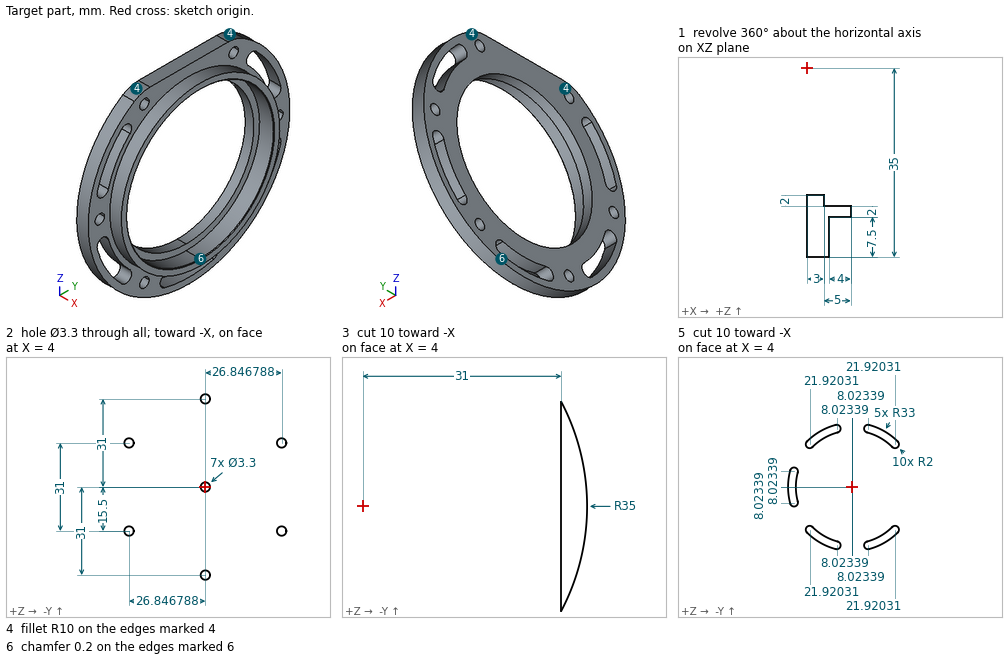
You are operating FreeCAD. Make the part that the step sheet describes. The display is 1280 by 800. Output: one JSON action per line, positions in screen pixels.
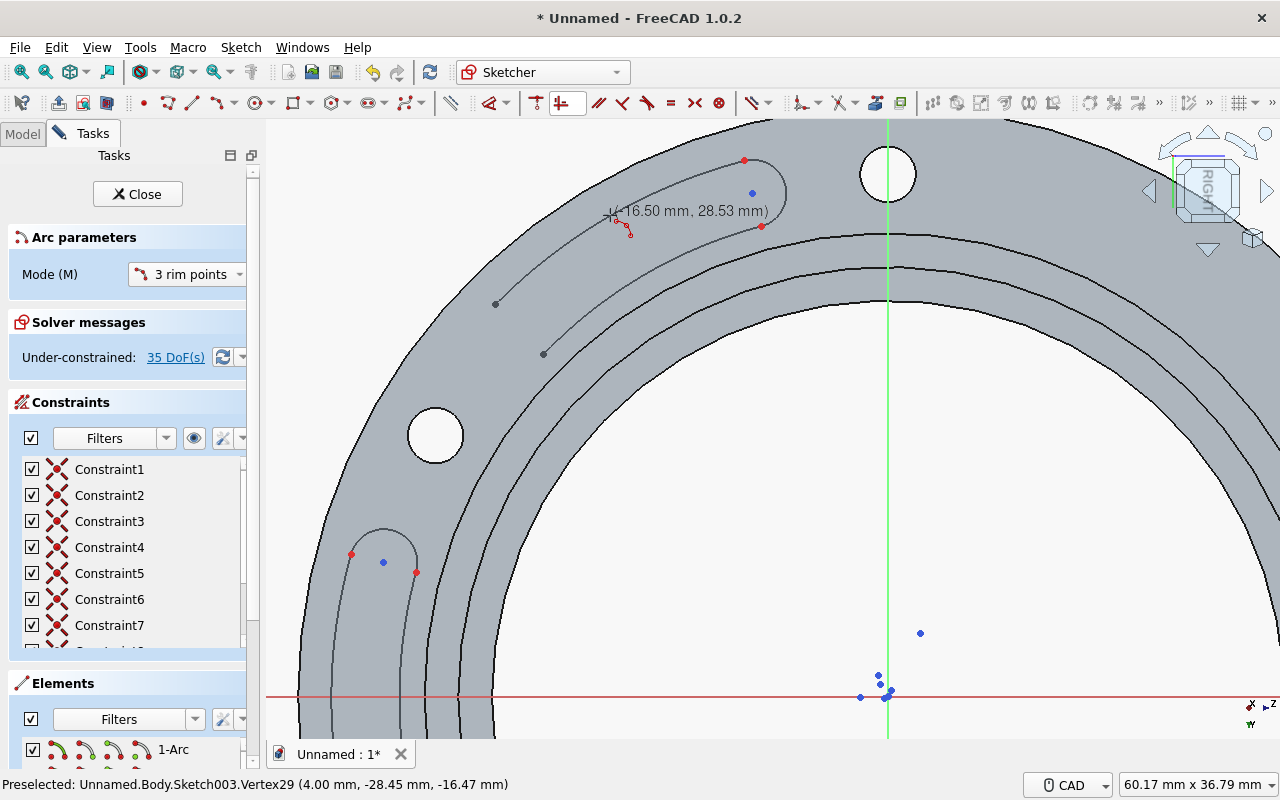
{"action": "left_click", "coordinate": [495, 305]}
{"action": "left_click", "coordinate": [544, 354]}
{"action": "left_click", "coordinate": [495, 351]}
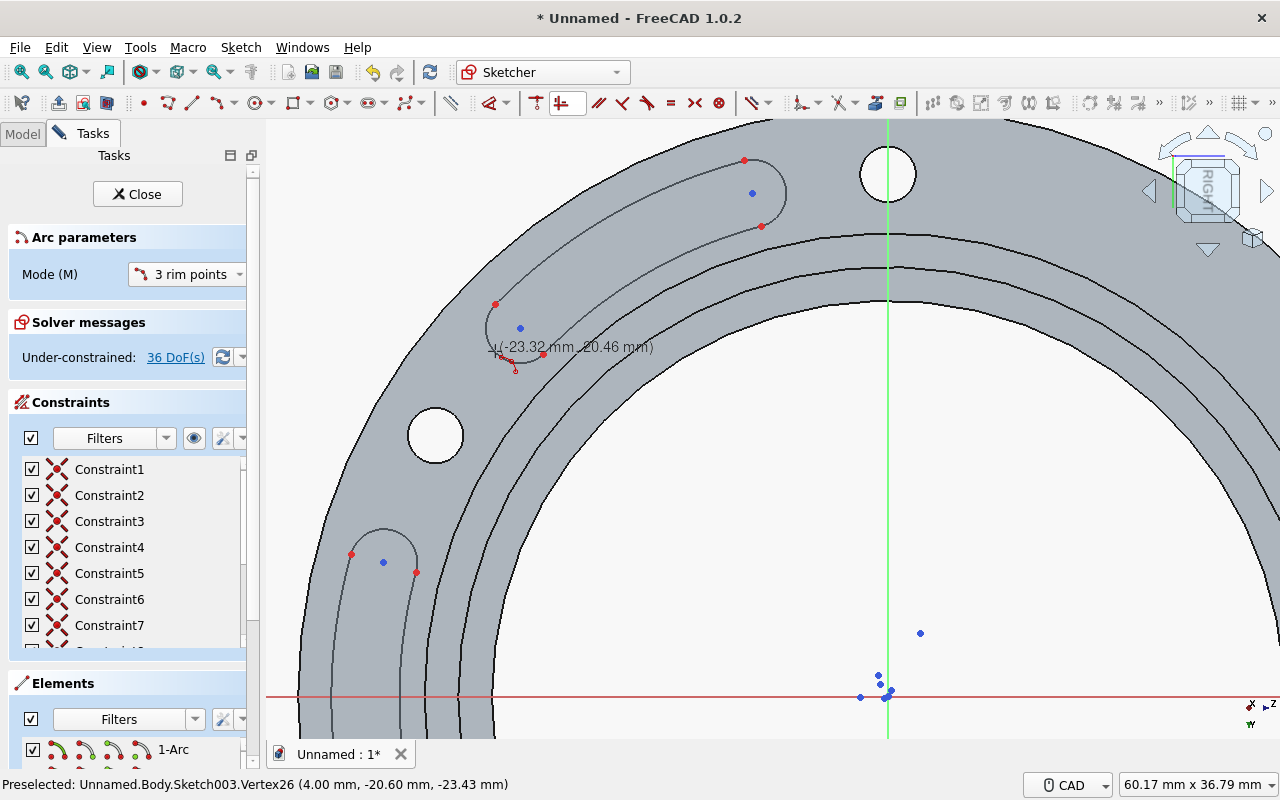
{"action": "scroll", "coordinate": [645, 273], "scroll_direction": "down", "scroll_amount": 5}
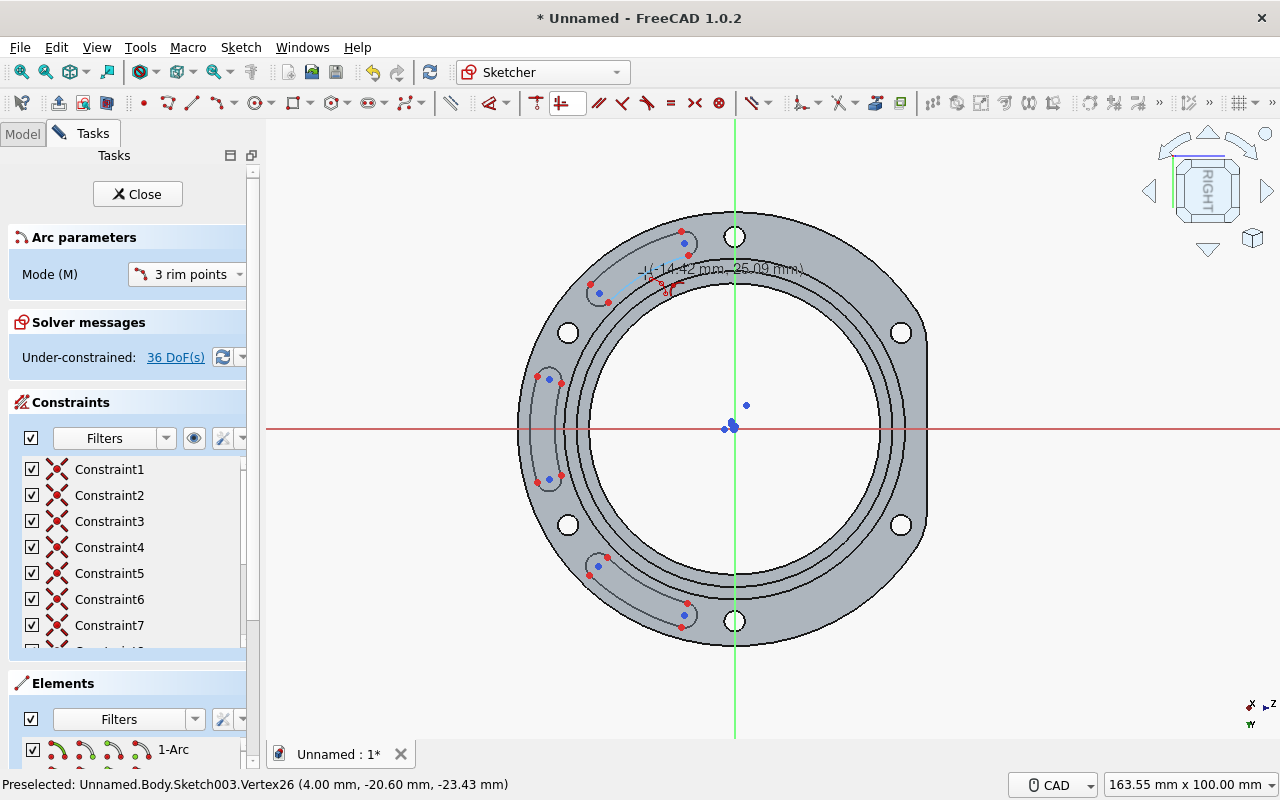
{"action": "left_click", "coordinate": [862, 302]}
{"action": "left_click", "coordinate": [879, 284]}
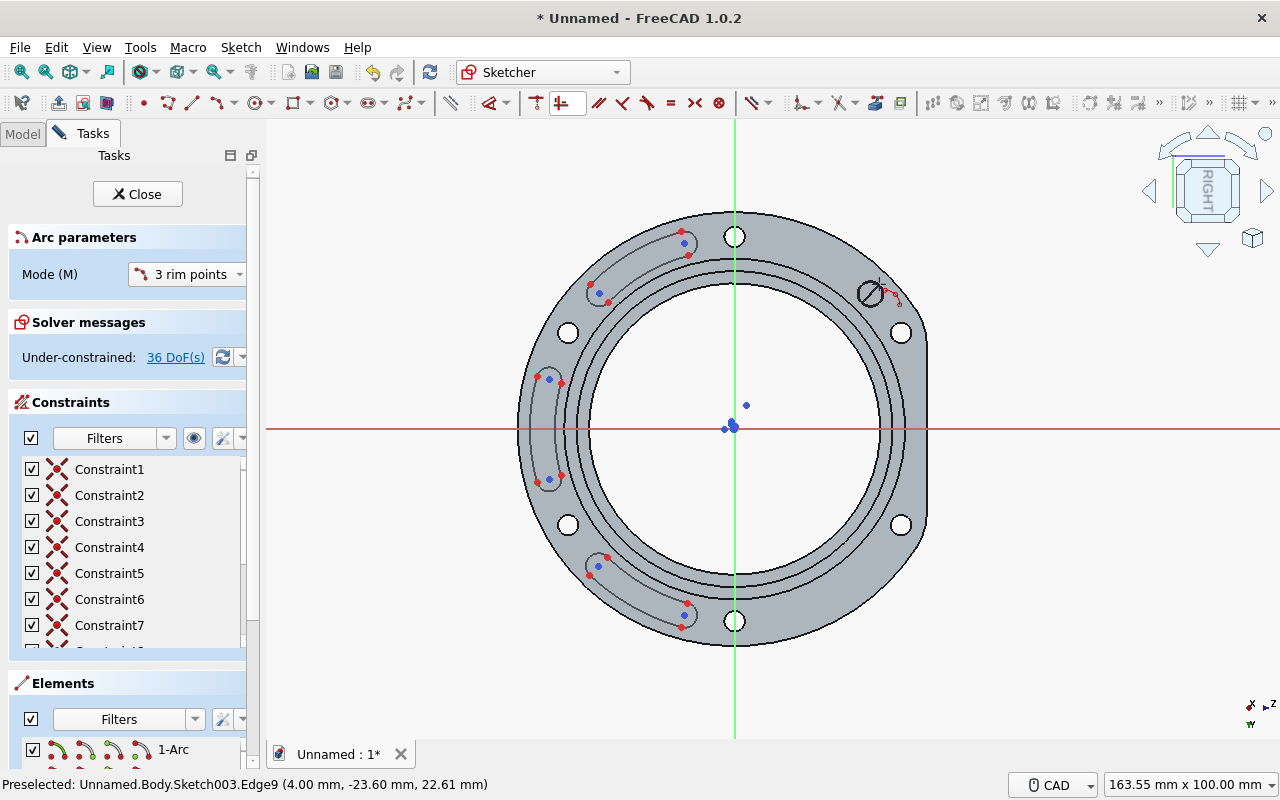
{"action": "scroll", "coordinate": [879, 302], "scroll_direction": "up", "scroll_amount": 2}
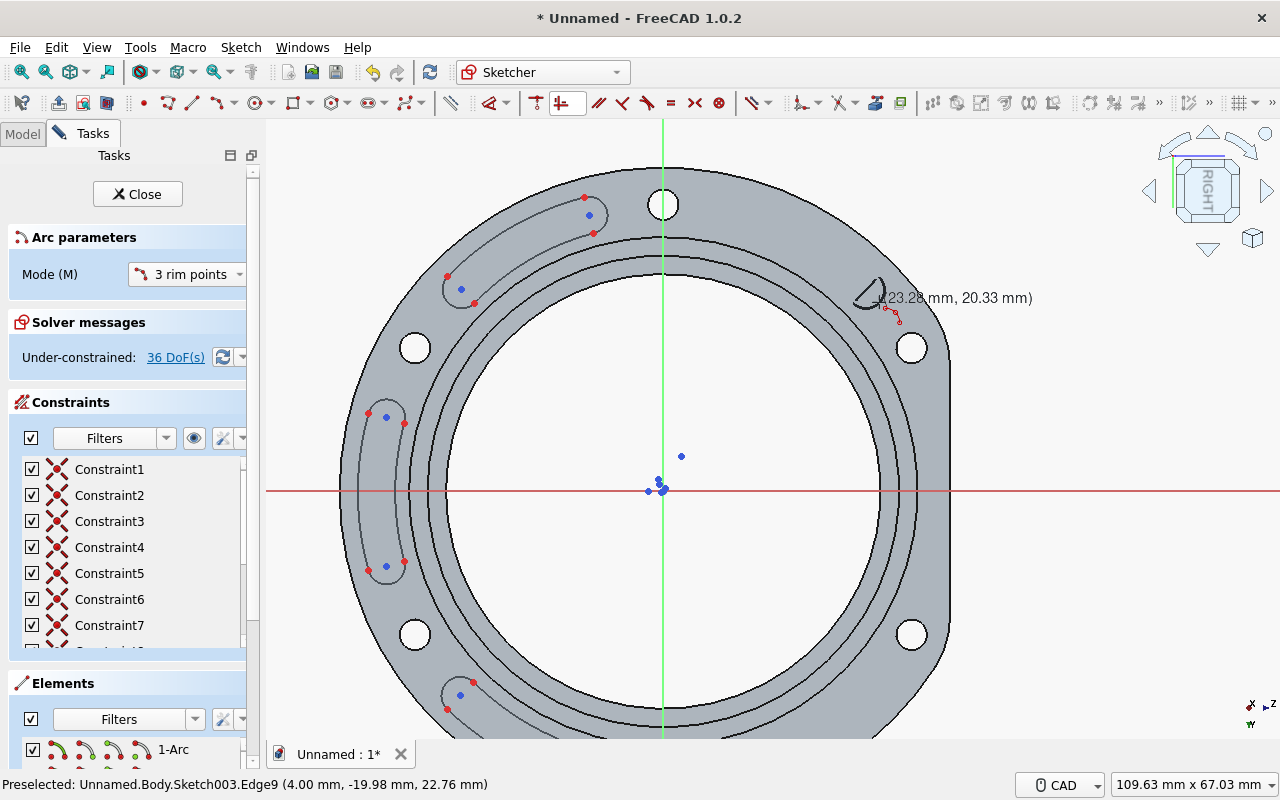
{"action": "left_click", "coordinate": [879, 302]}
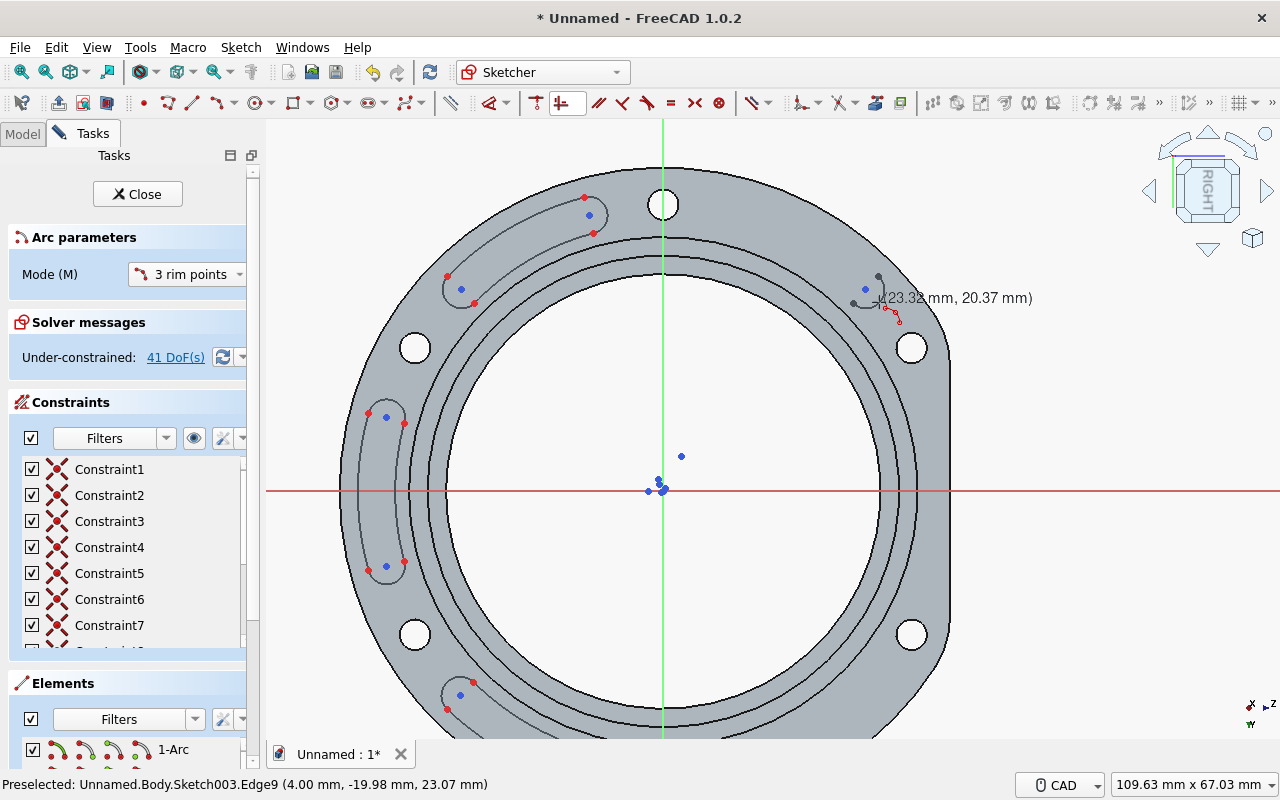
{"action": "left_click", "coordinate": [879, 276]}
{"action": "left_click", "coordinate": [742, 197]}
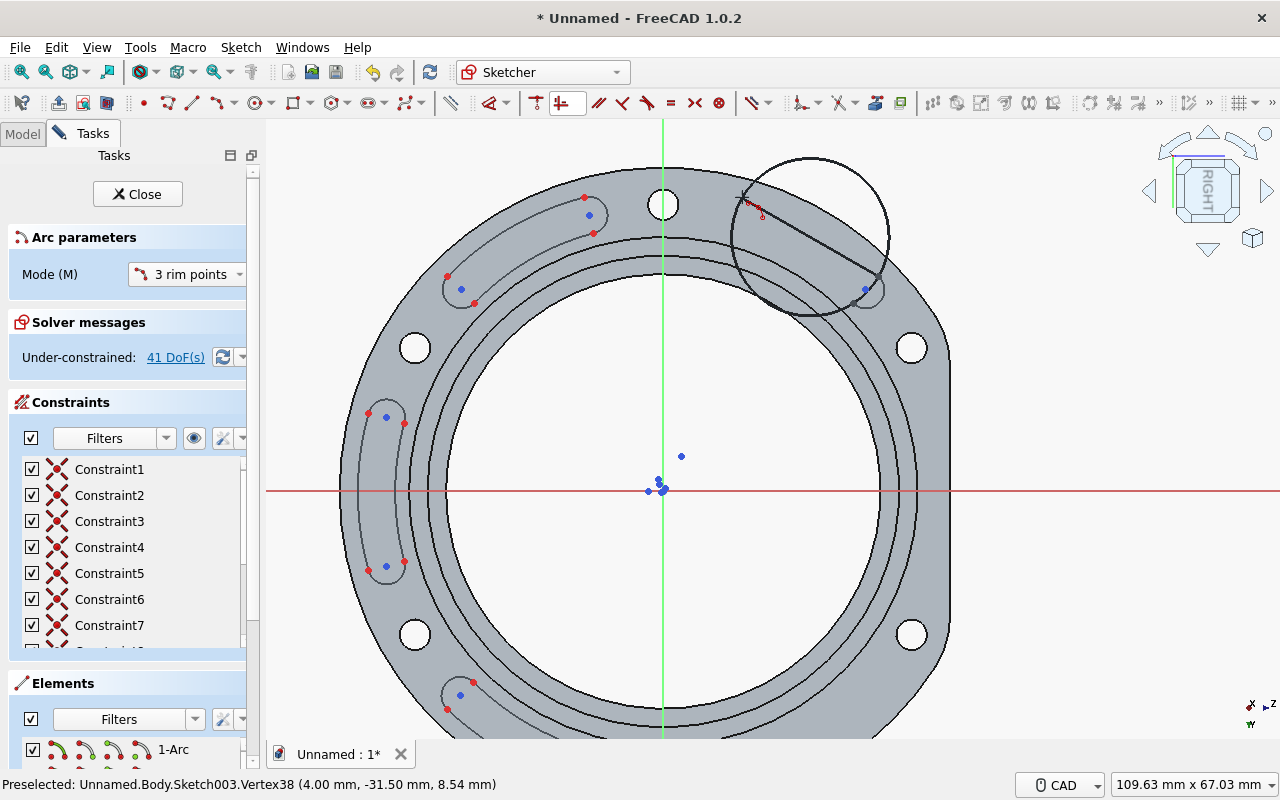
{"action": "scroll", "coordinate": [816, 227], "scroll_direction": "up", "scroll_amount": 3}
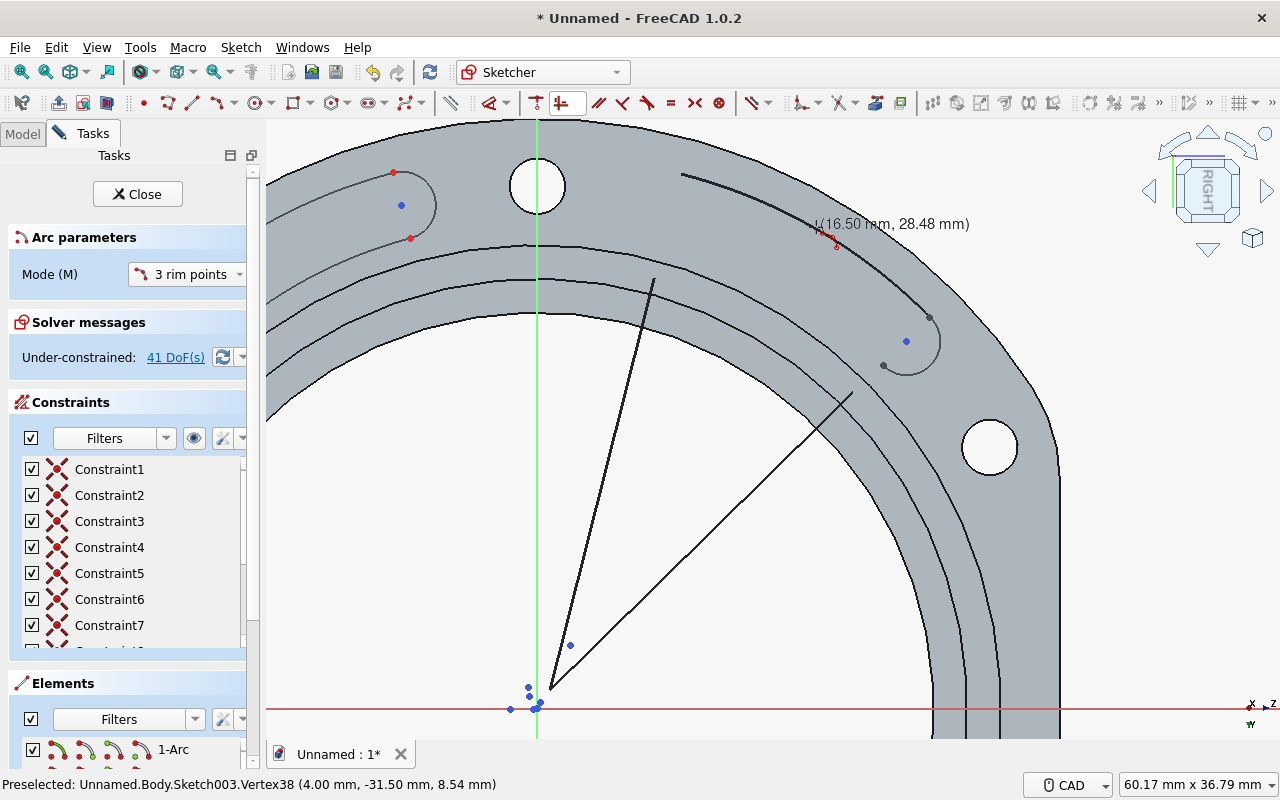
{"action": "left_click", "coordinate": [815, 227]}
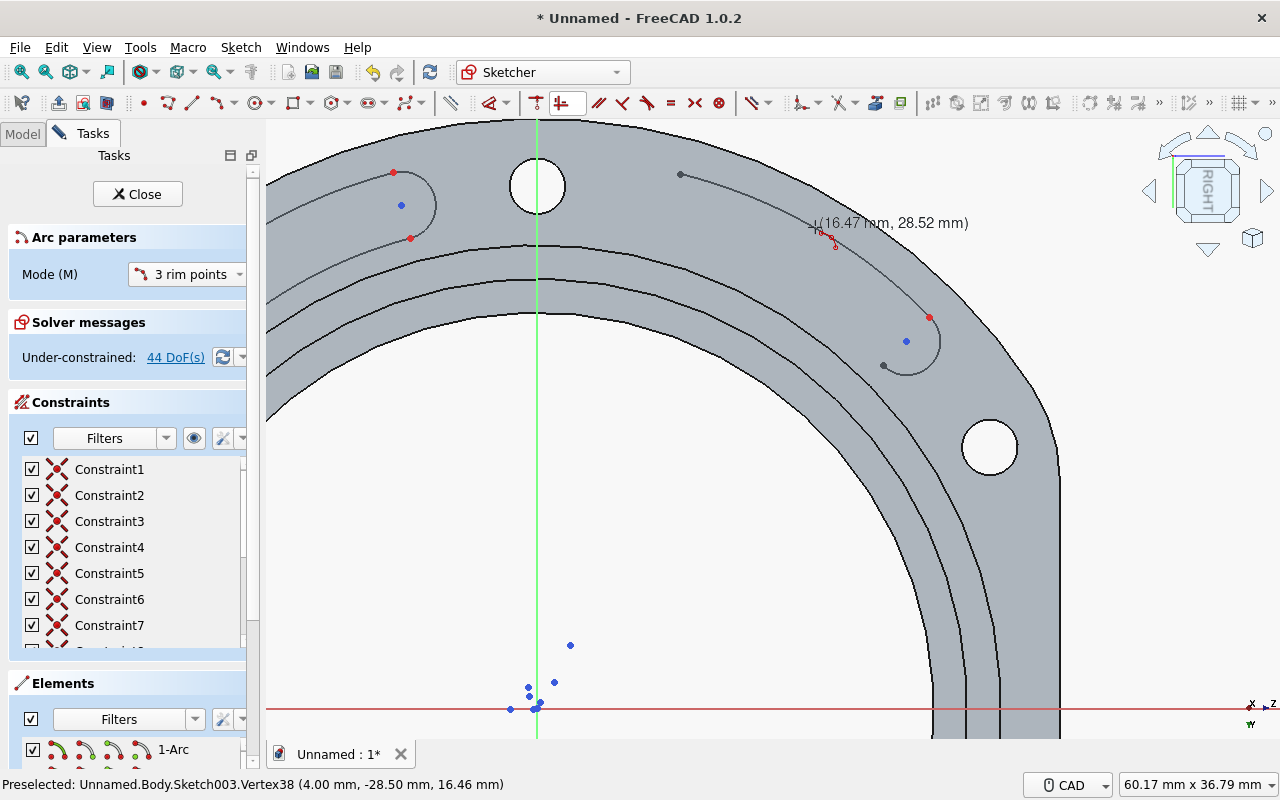
{"action": "left_click", "coordinate": [681, 174]}
{"action": "left_click", "coordinate": [664, 237]}
{"action": "left_click", "coordinate": [640, 195]}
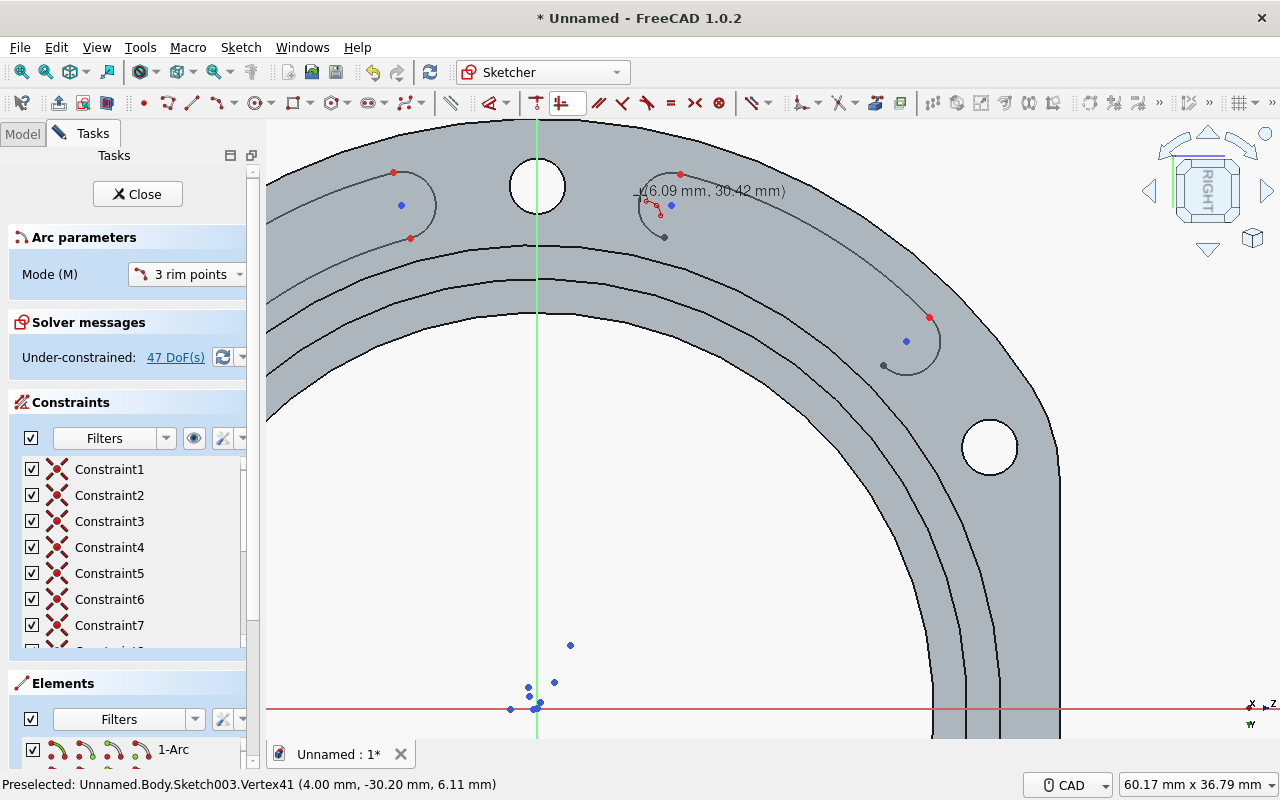
{"action": "left_click", "coordinate": [664, 238]}
{"action": "left_click", "coordinate": [884, 366]}
{"action": "left_click", "coordinate": [782, 285]}